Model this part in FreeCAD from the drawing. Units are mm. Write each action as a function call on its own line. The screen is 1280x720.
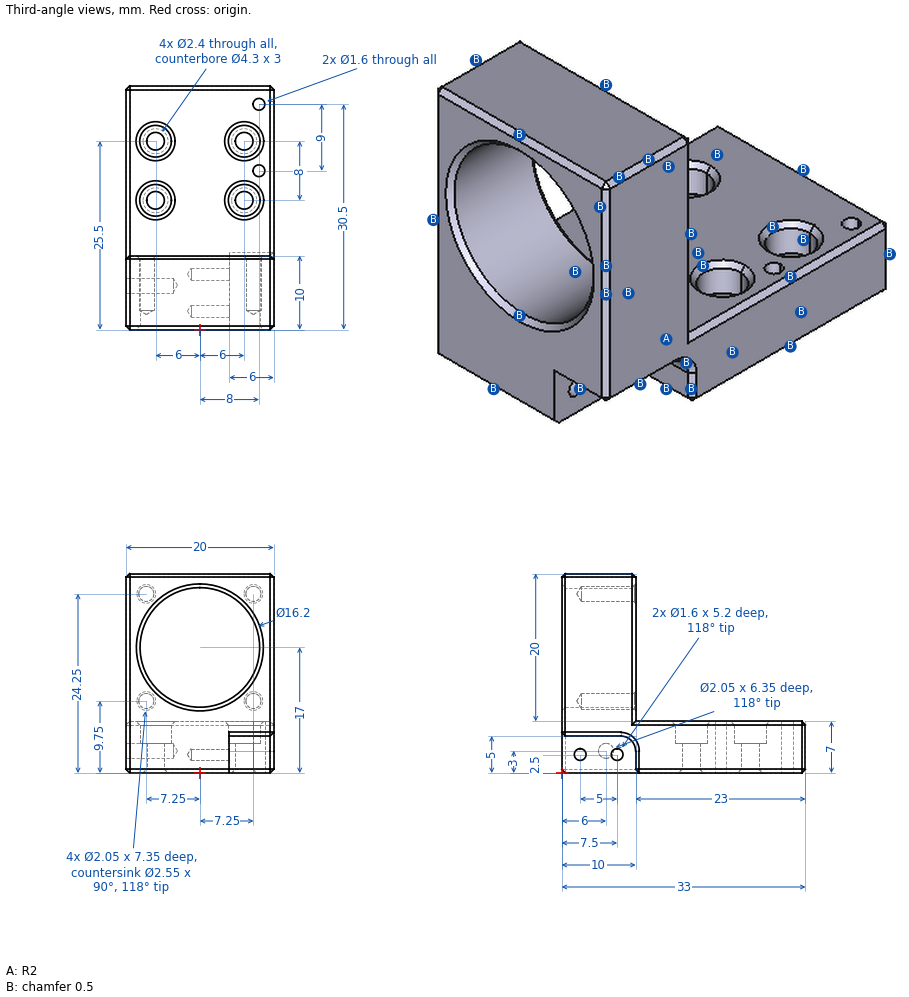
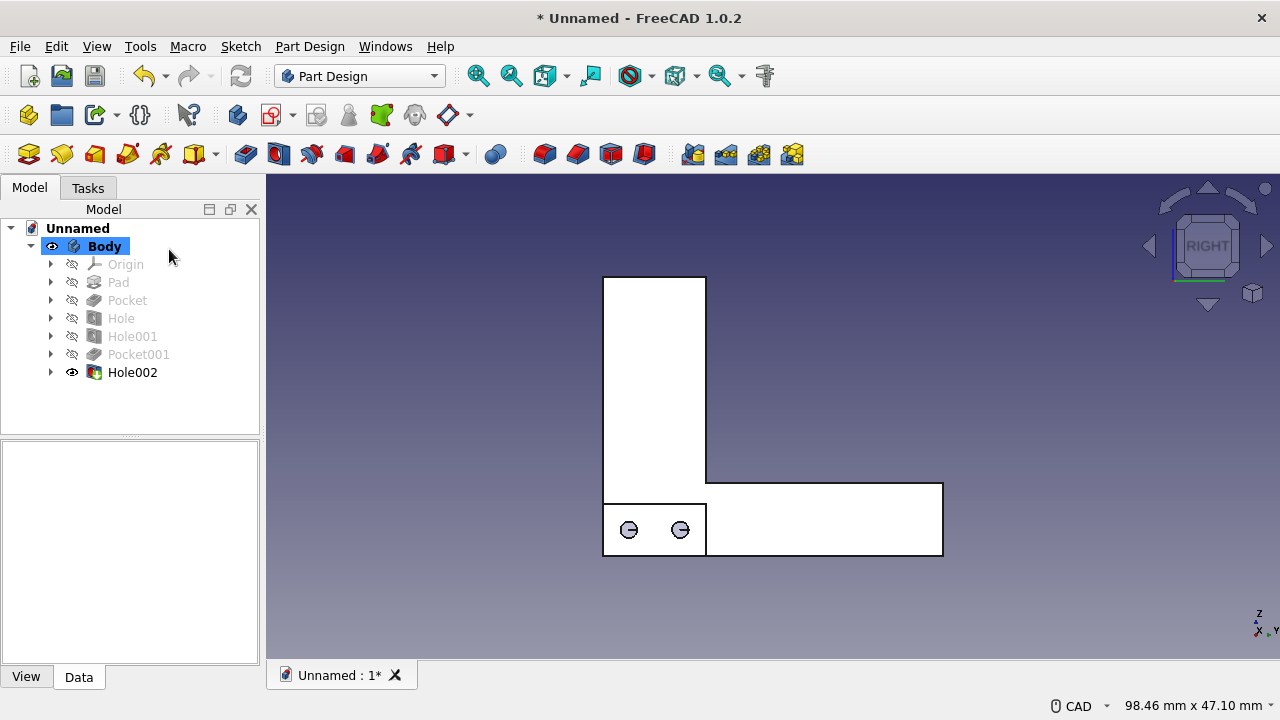
key(0)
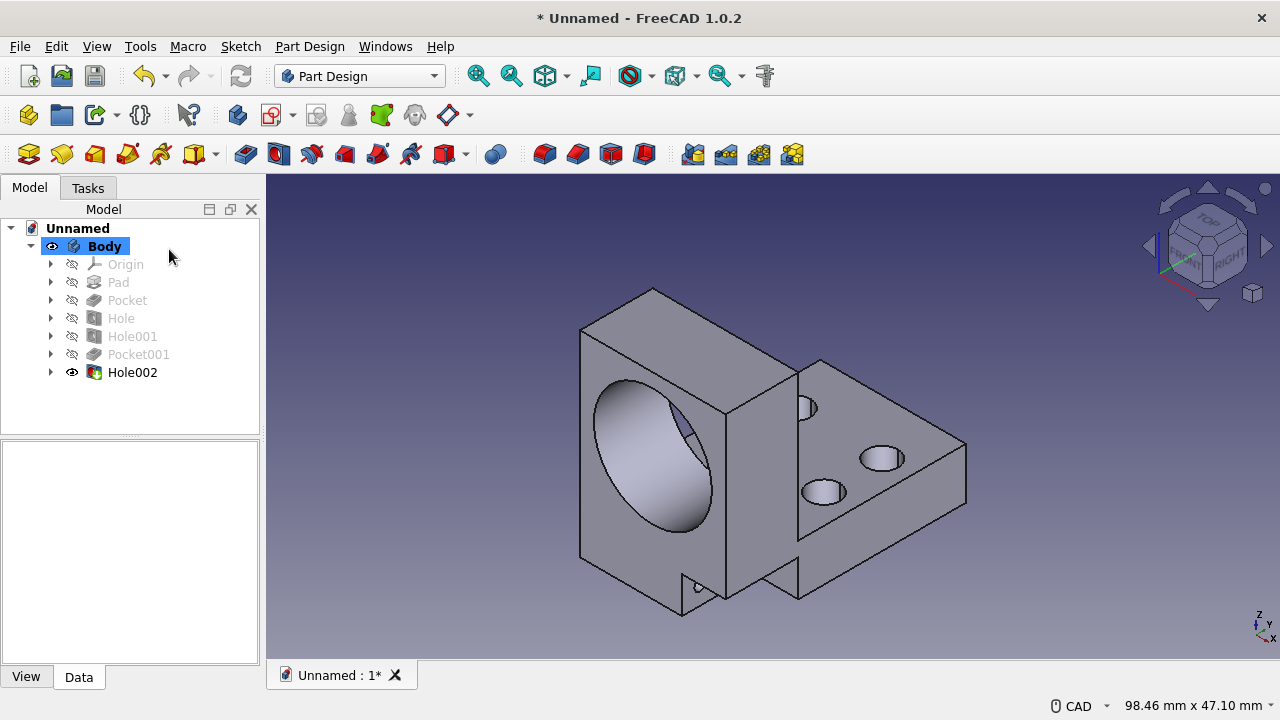
key(2)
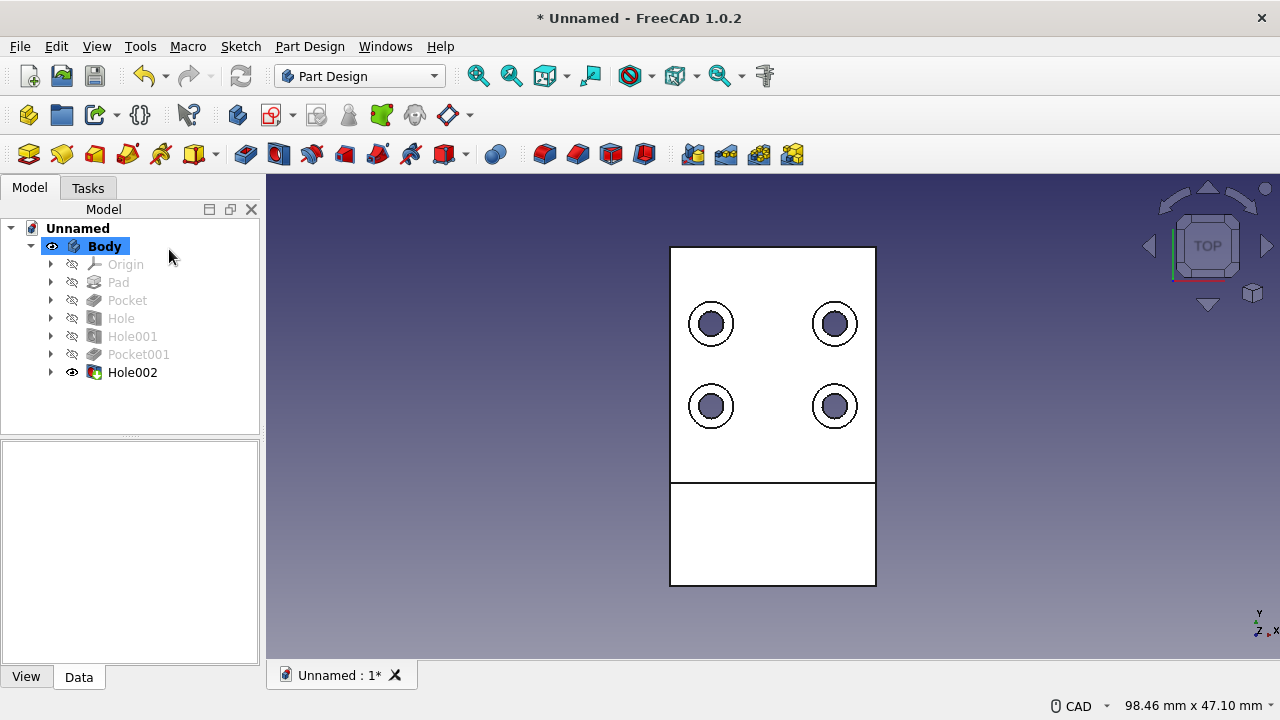
key(1)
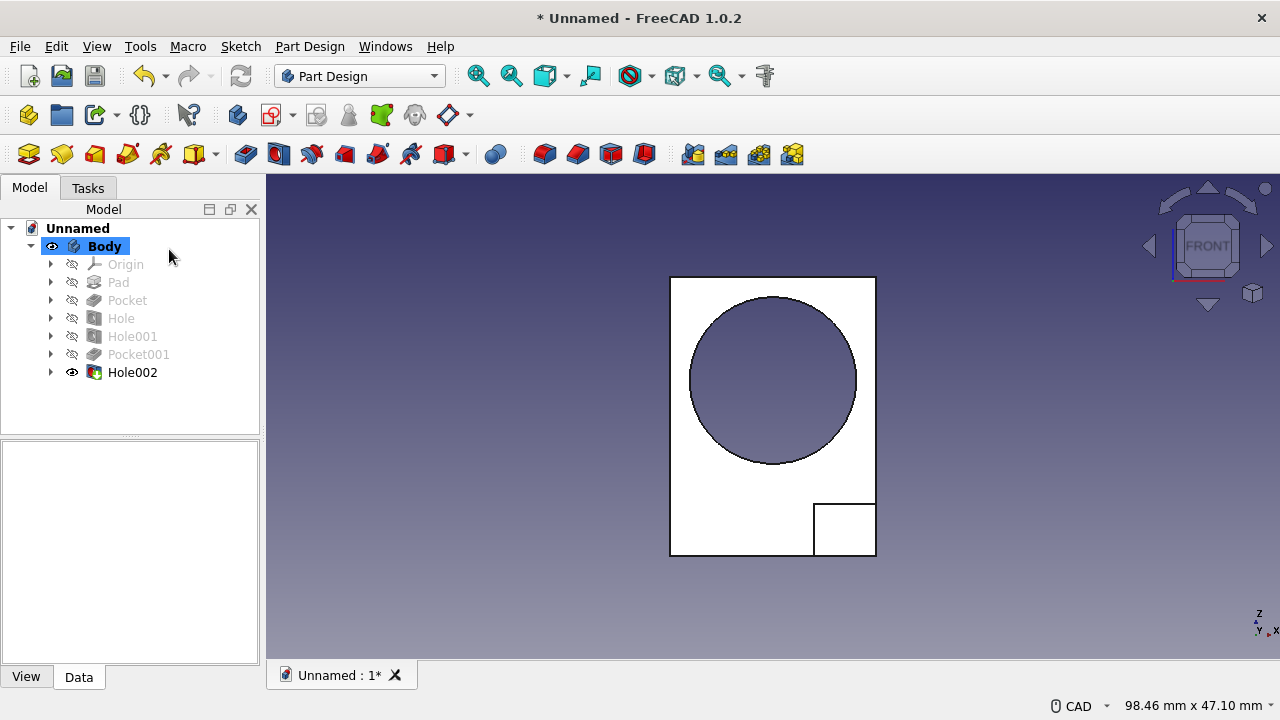
key(3)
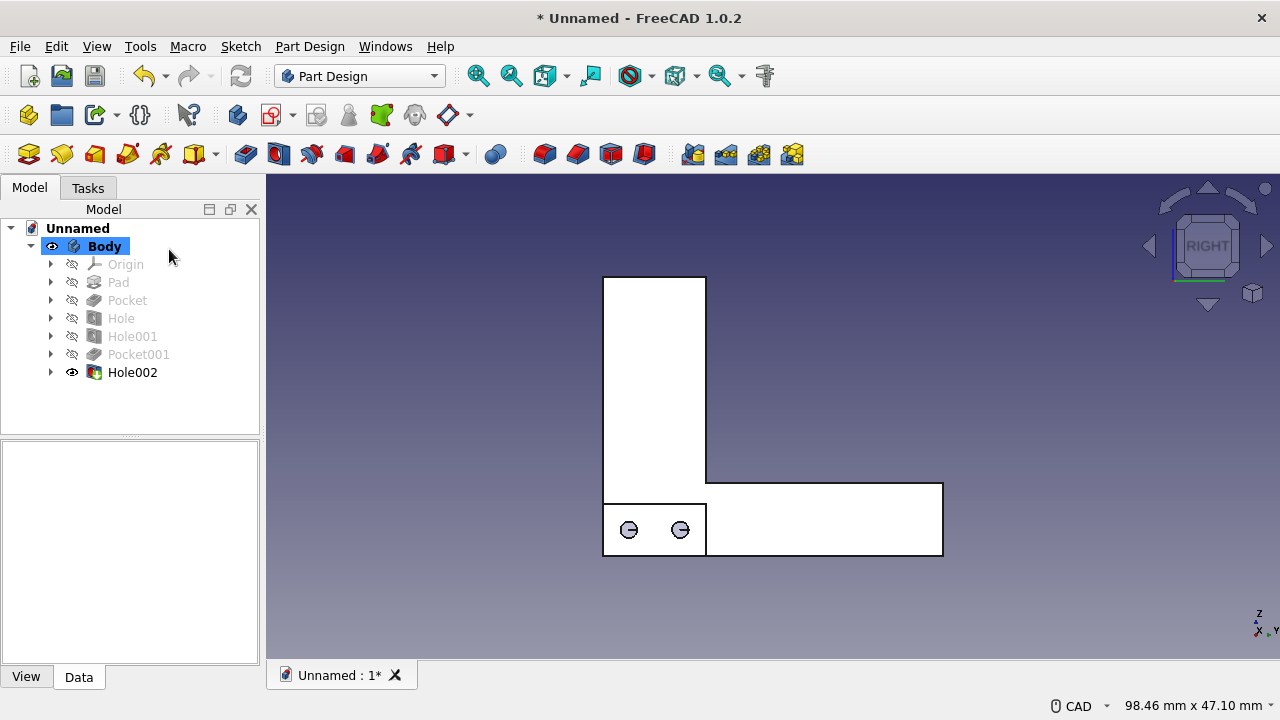
key(5)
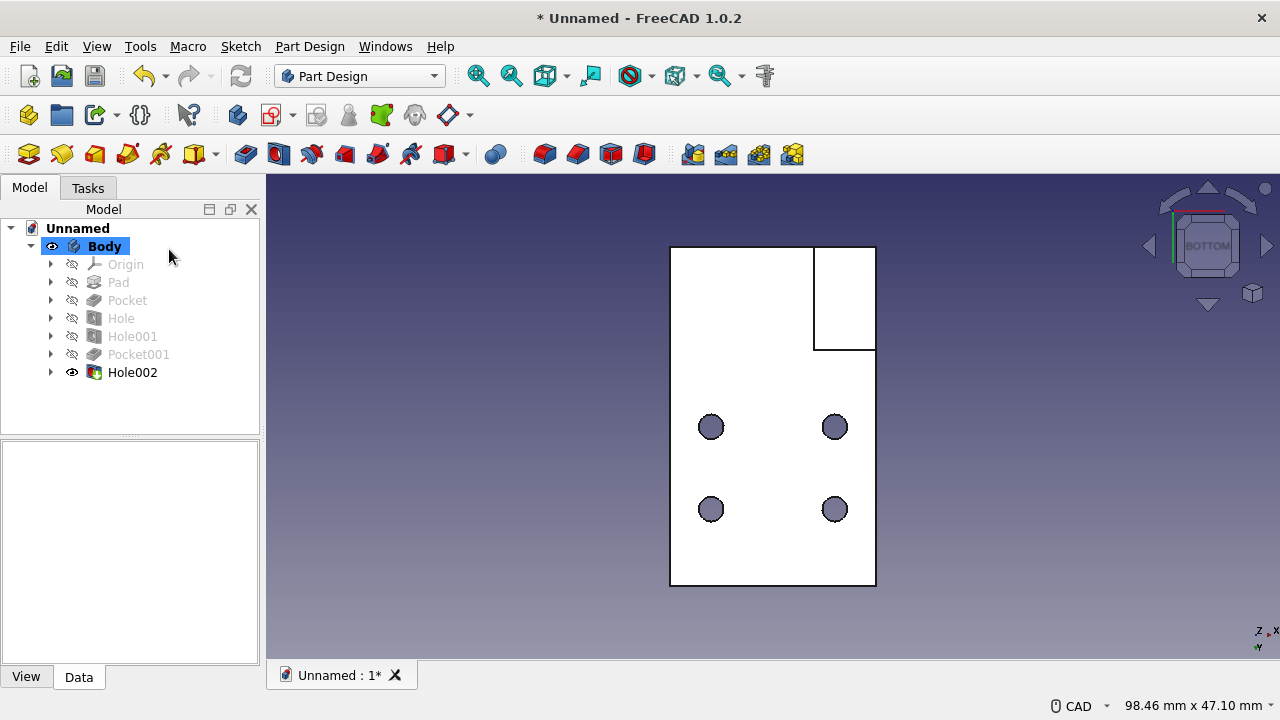
key(4)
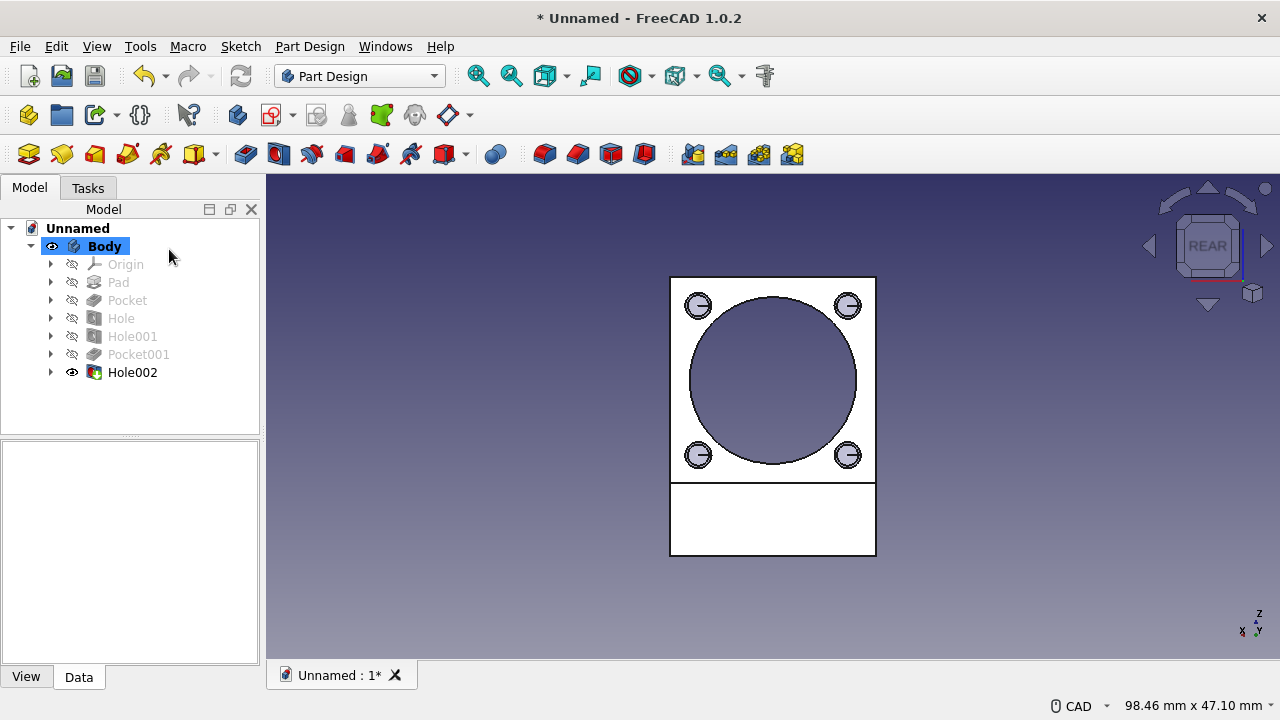
key(6)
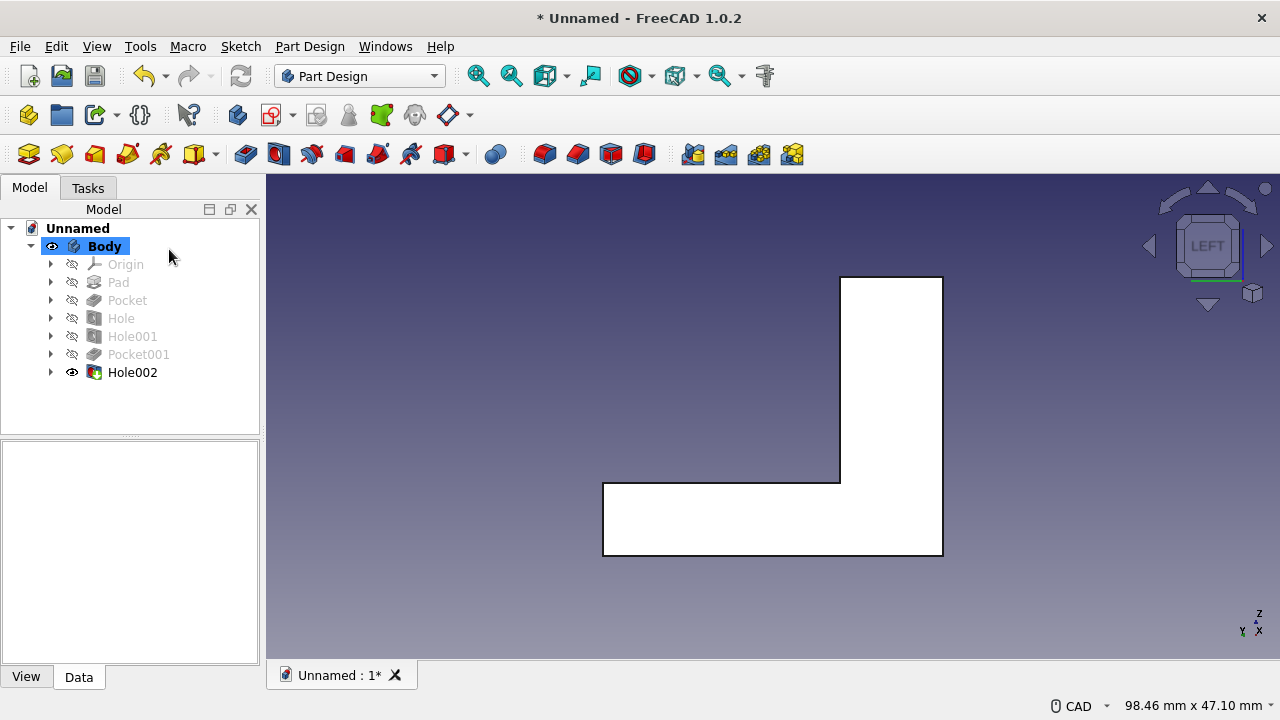
key(v)
key(3)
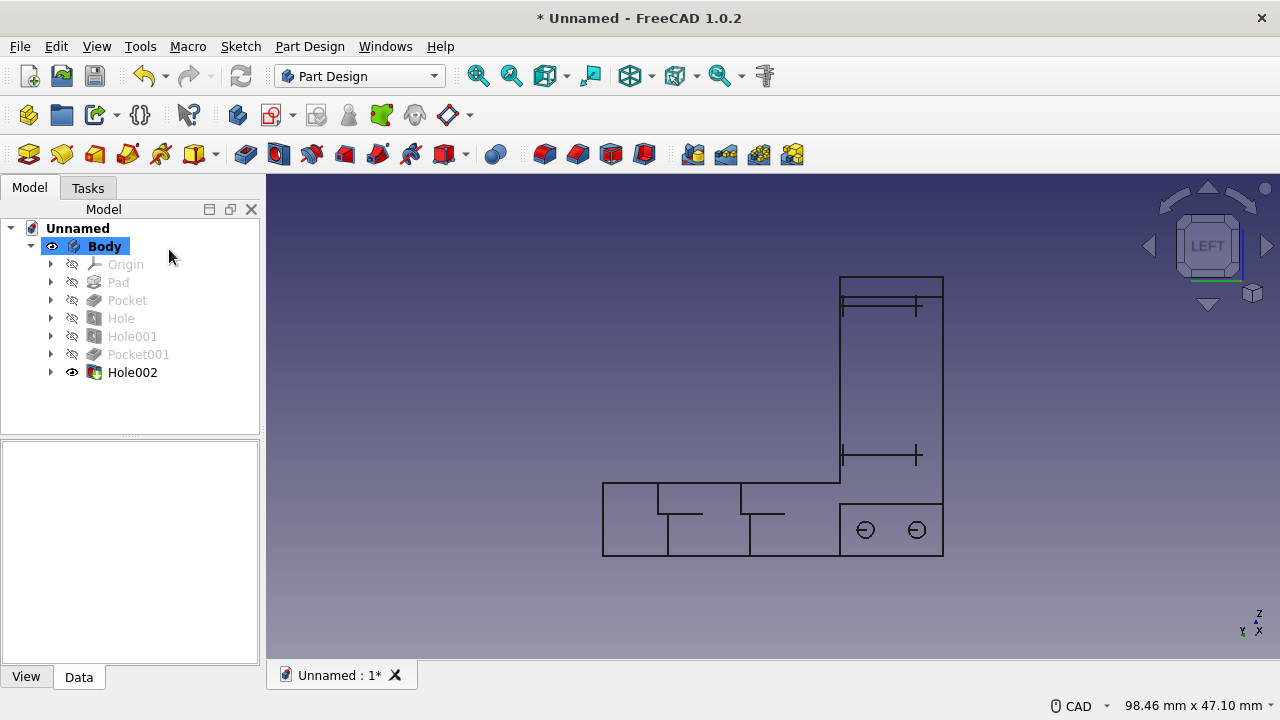
key(0)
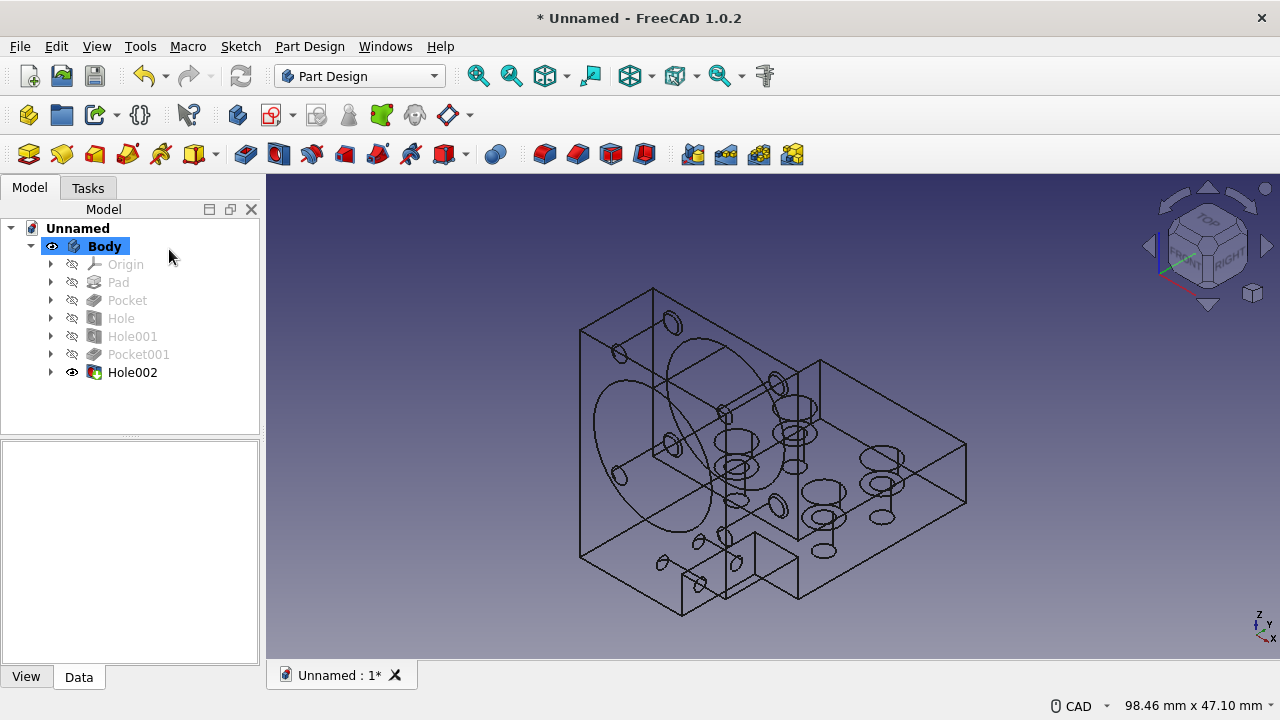
click(777, 544)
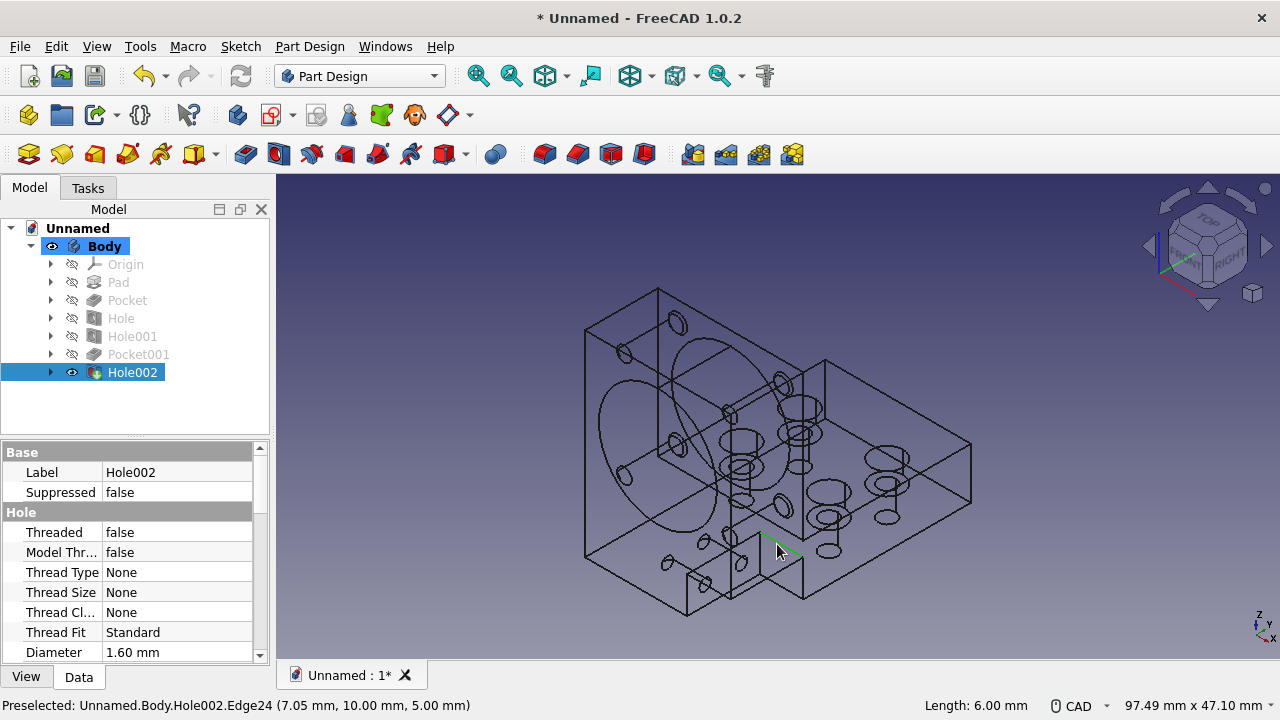
key(v)
key(1)